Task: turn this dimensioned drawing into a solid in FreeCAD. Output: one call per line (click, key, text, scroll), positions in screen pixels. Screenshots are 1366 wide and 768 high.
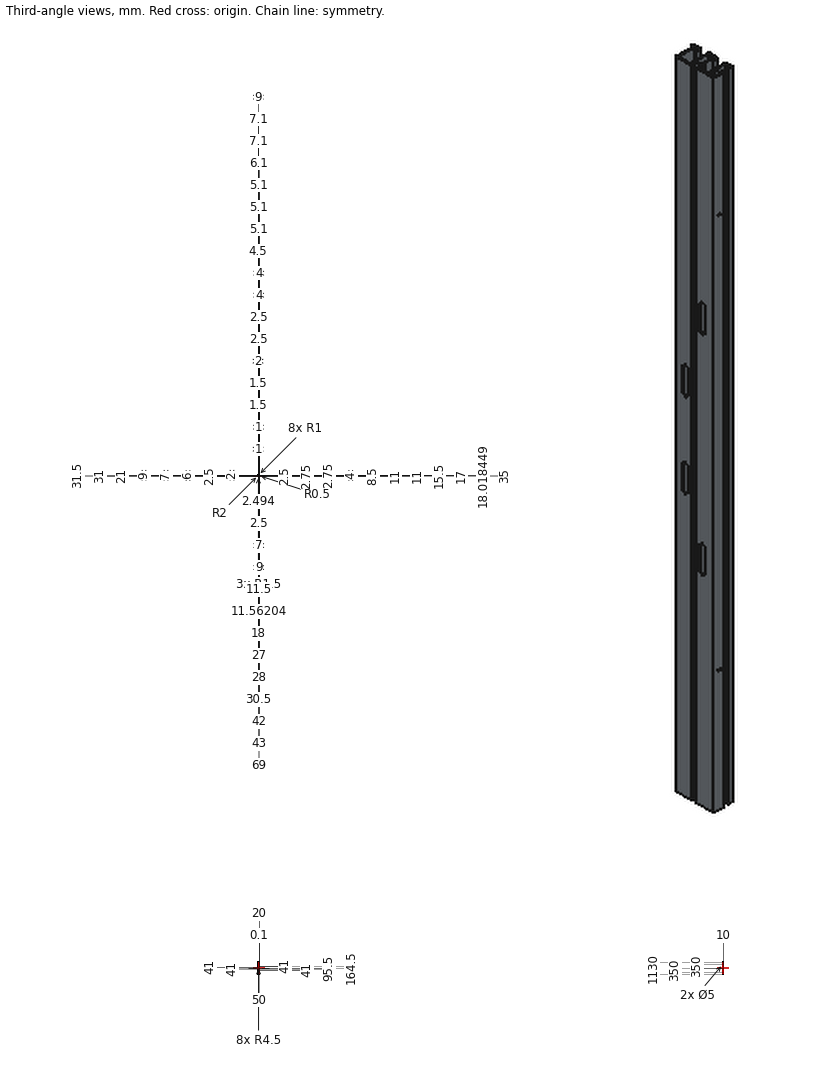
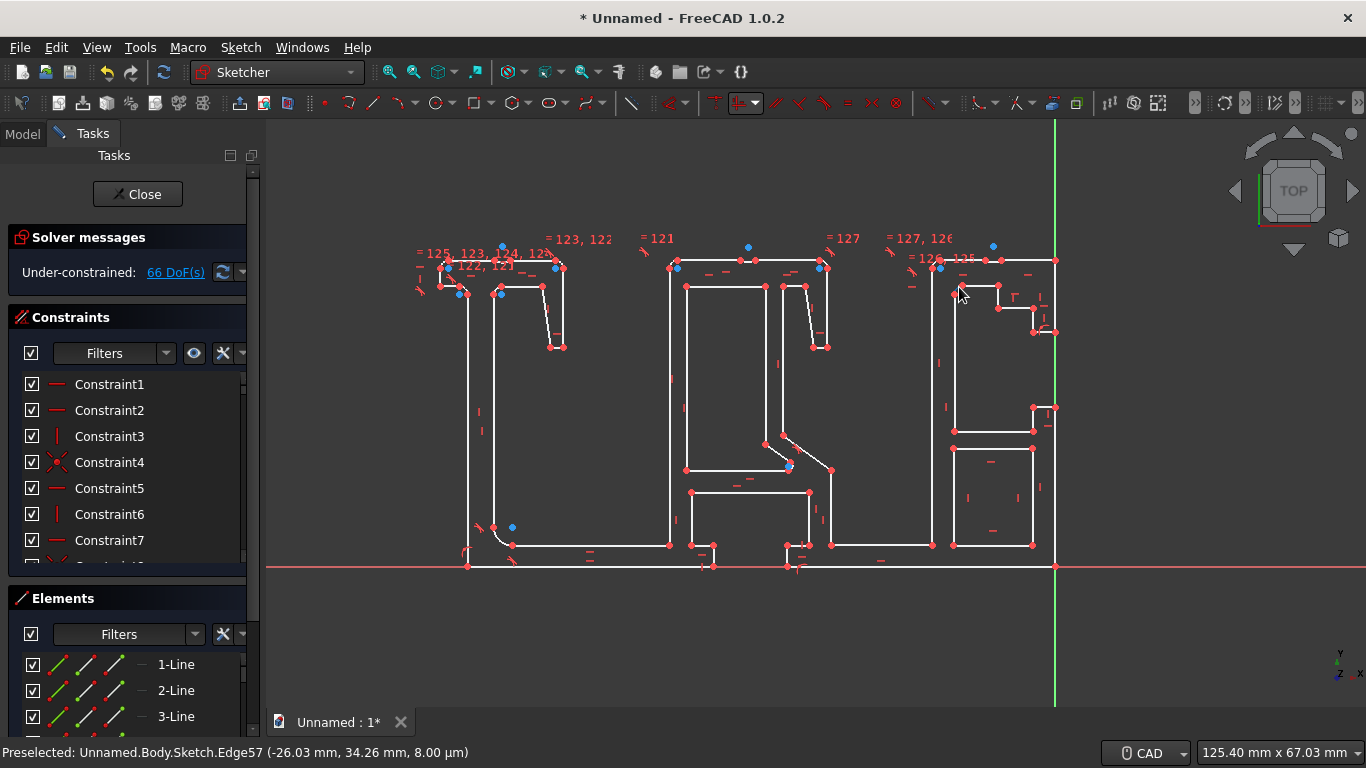
scroll(745, 262, up, 6)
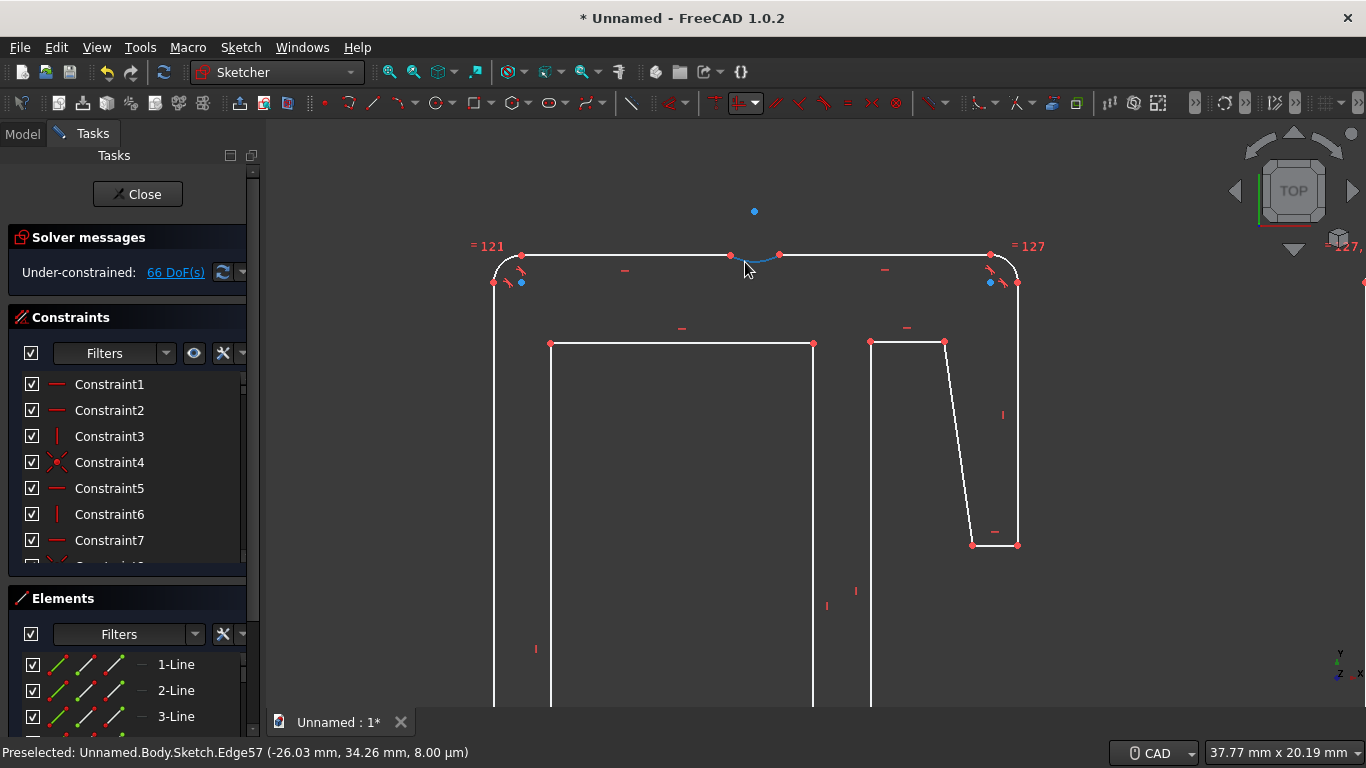
click(745, 261)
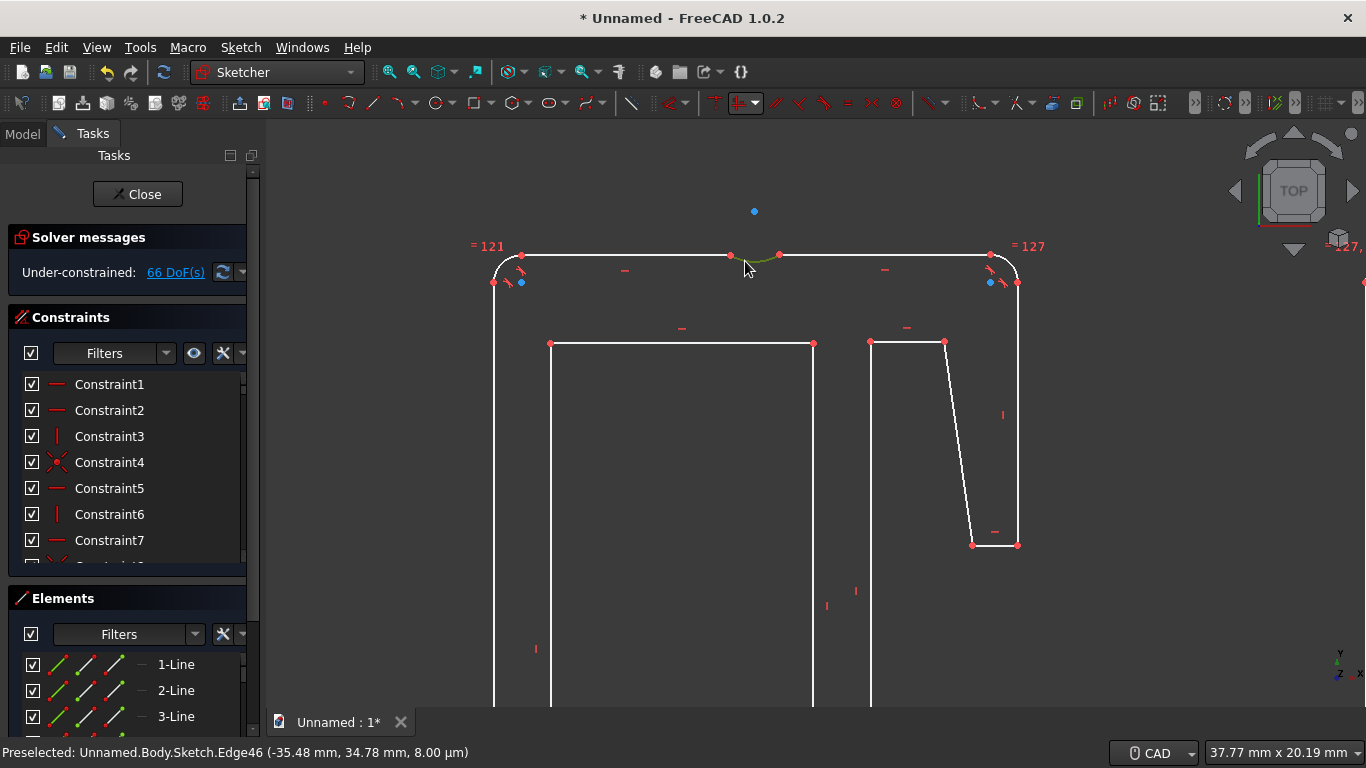
scroll(744, 262, down, 6)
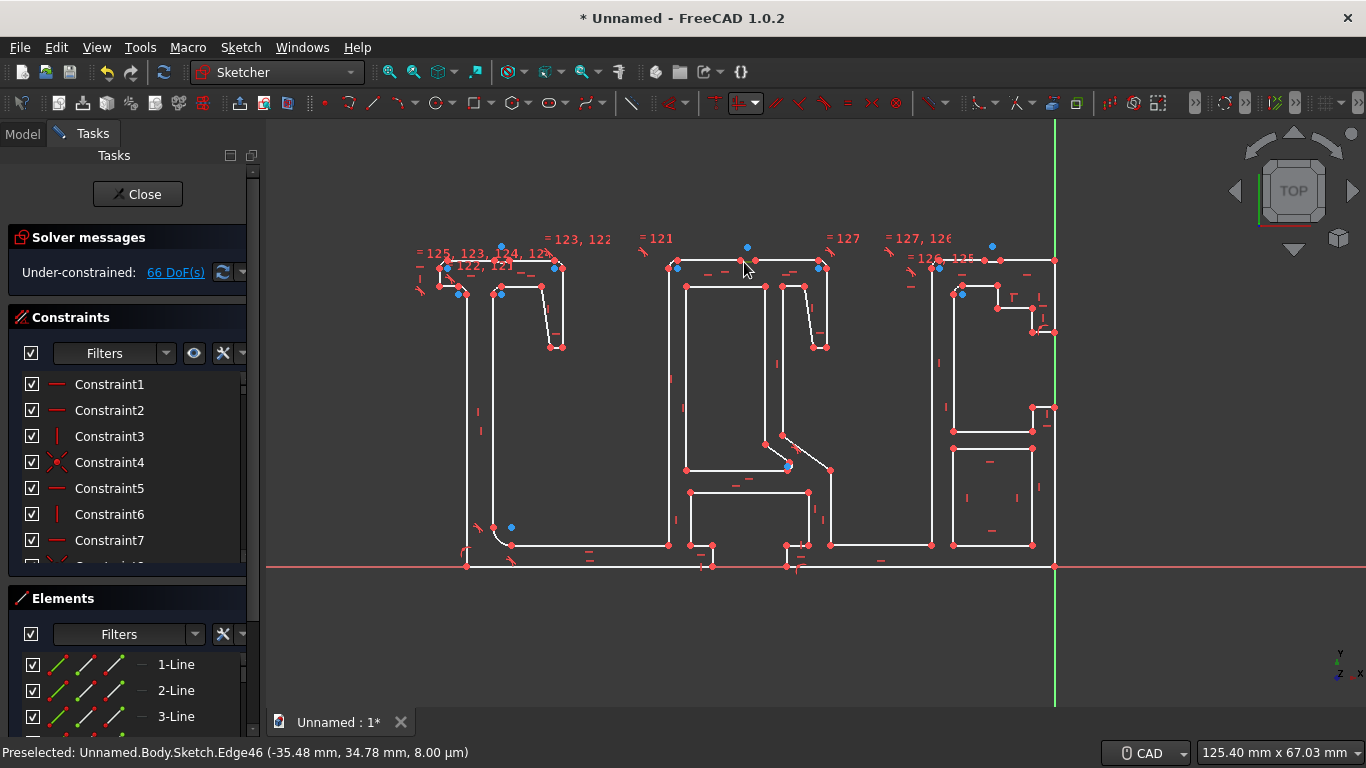
scroll(499, 262, up, 6)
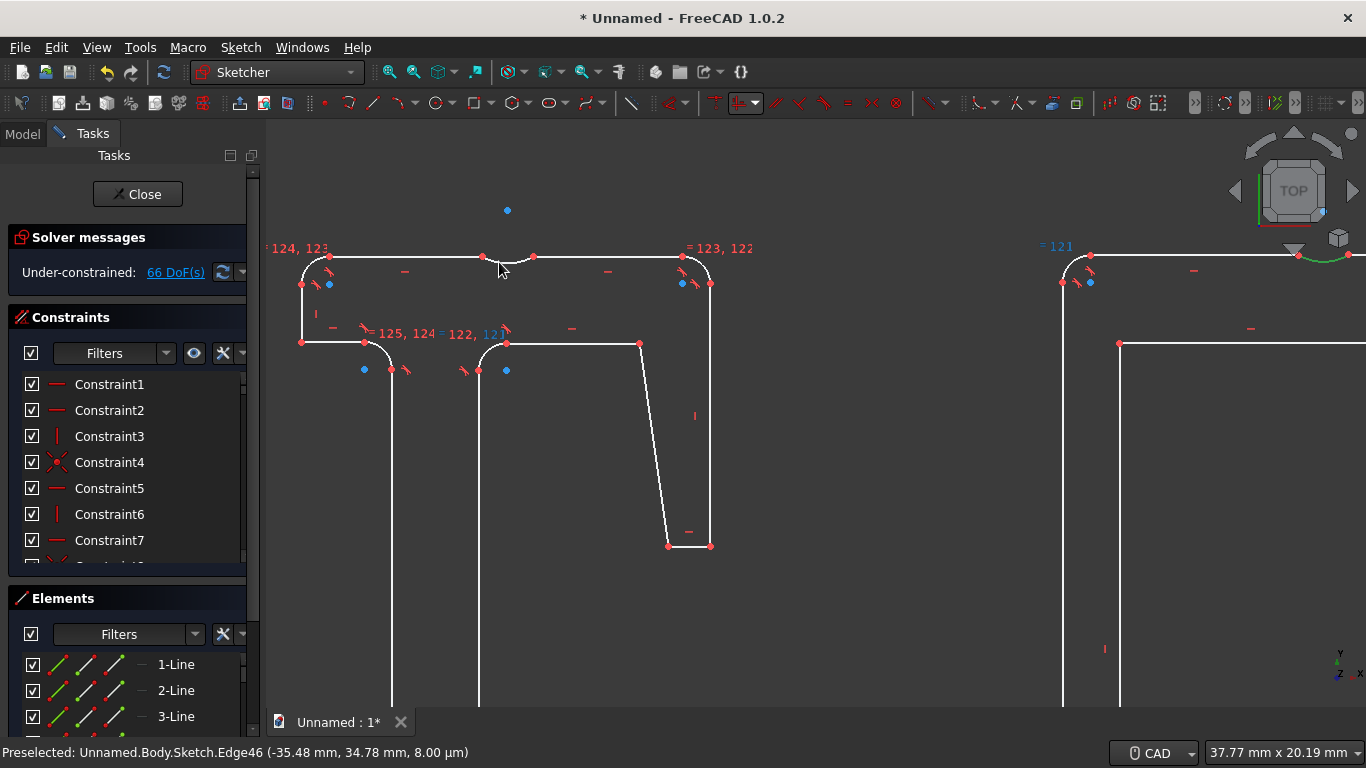
click(497, 262)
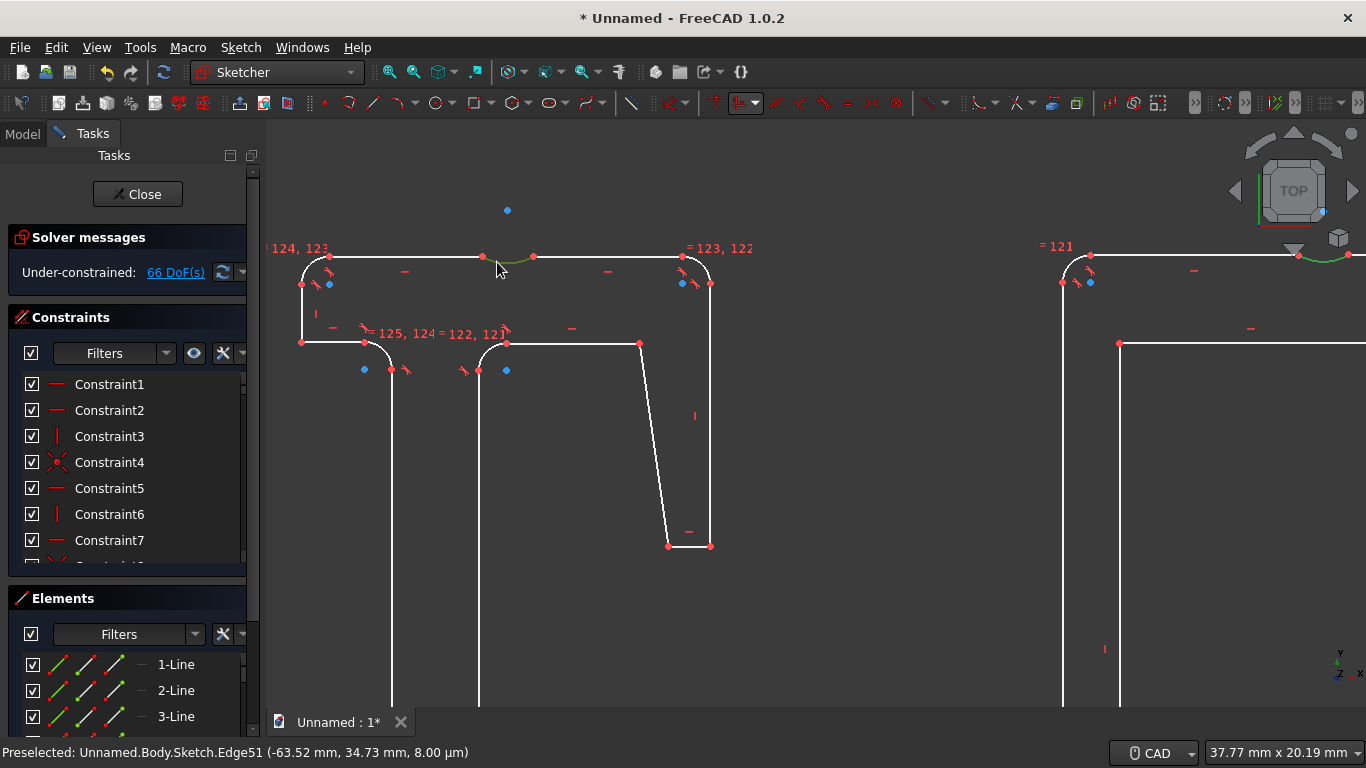
scroll(499, 262, down, 6)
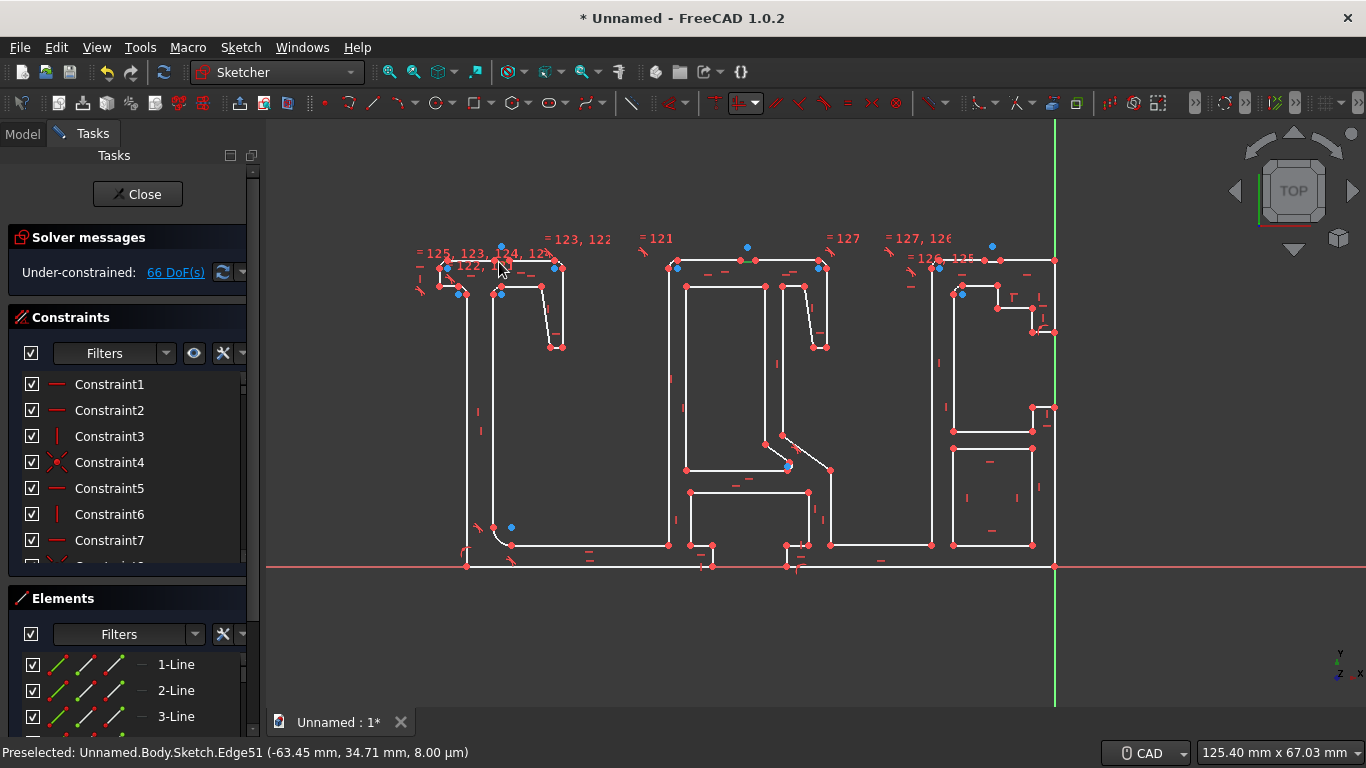
scroll(990, 262, up, 6)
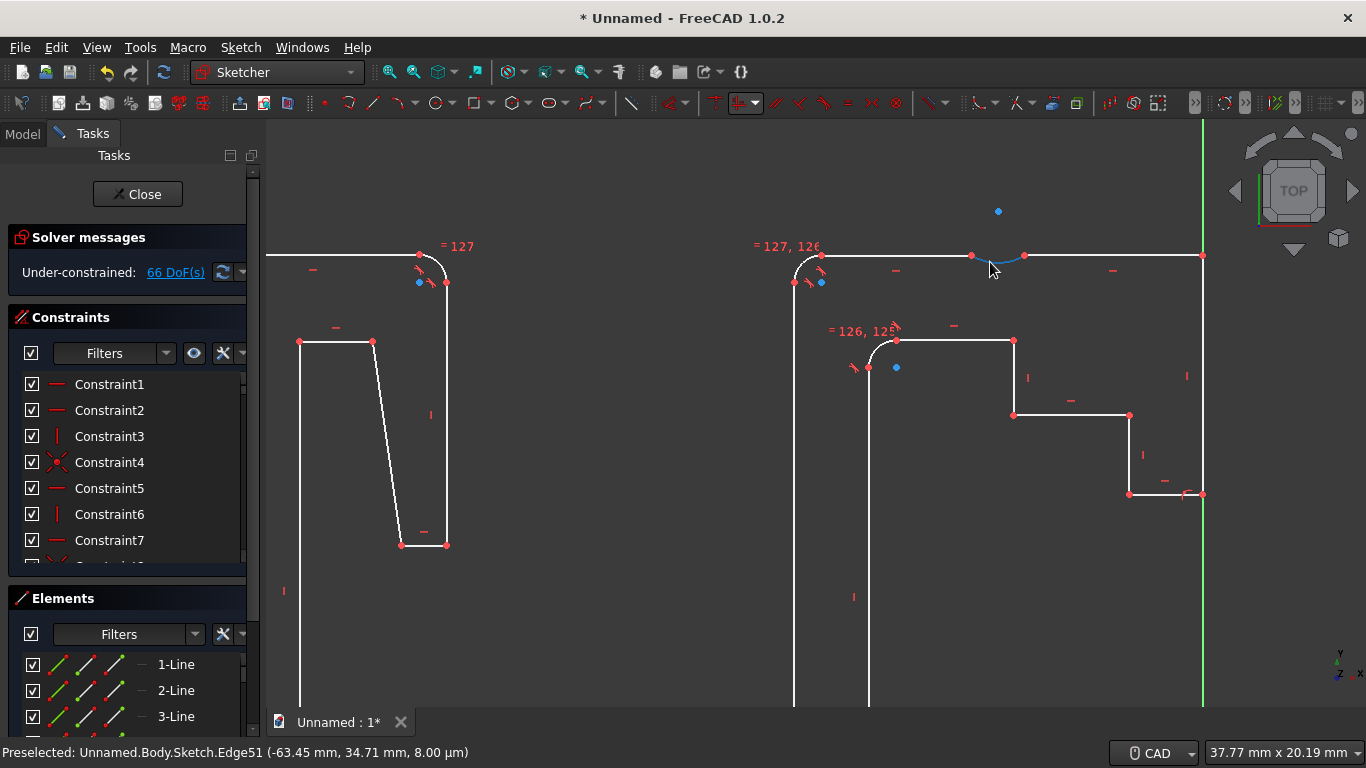
click(987, 262)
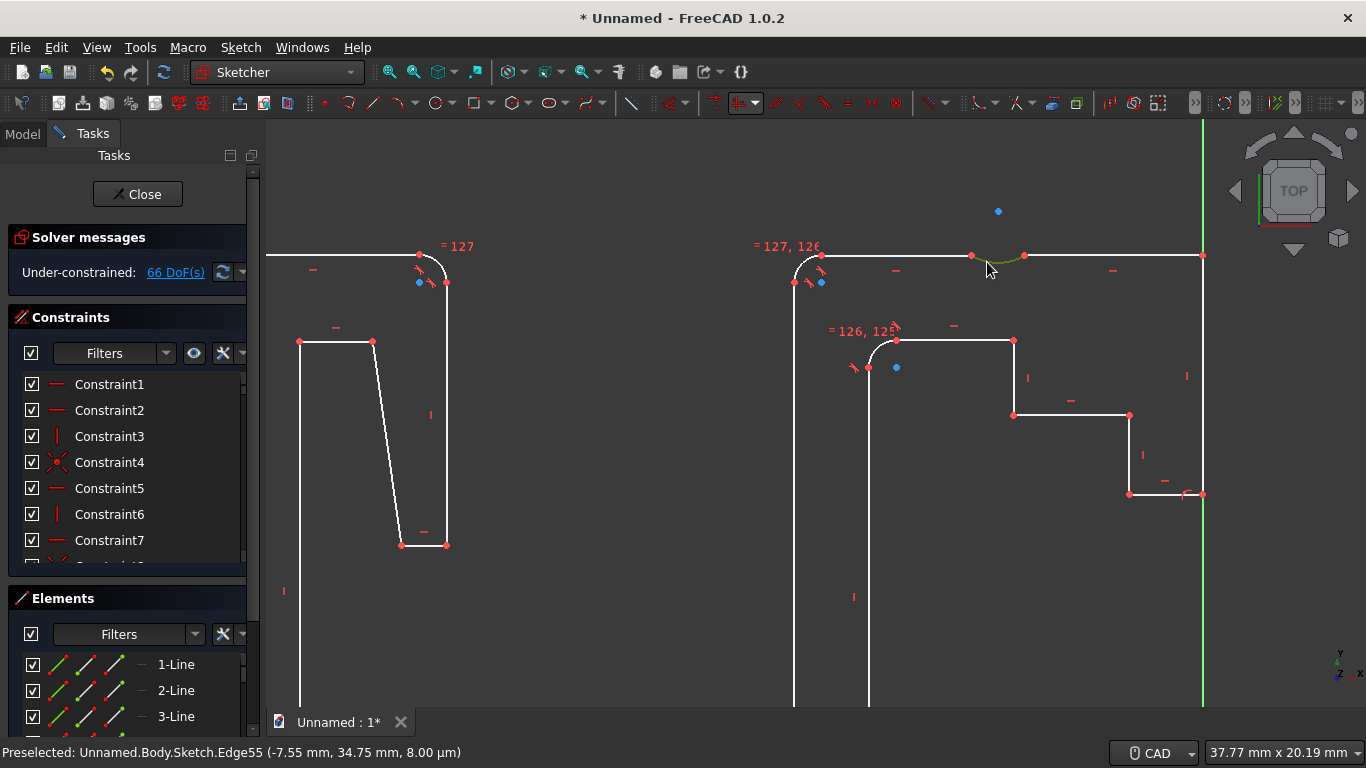
click(848, 104)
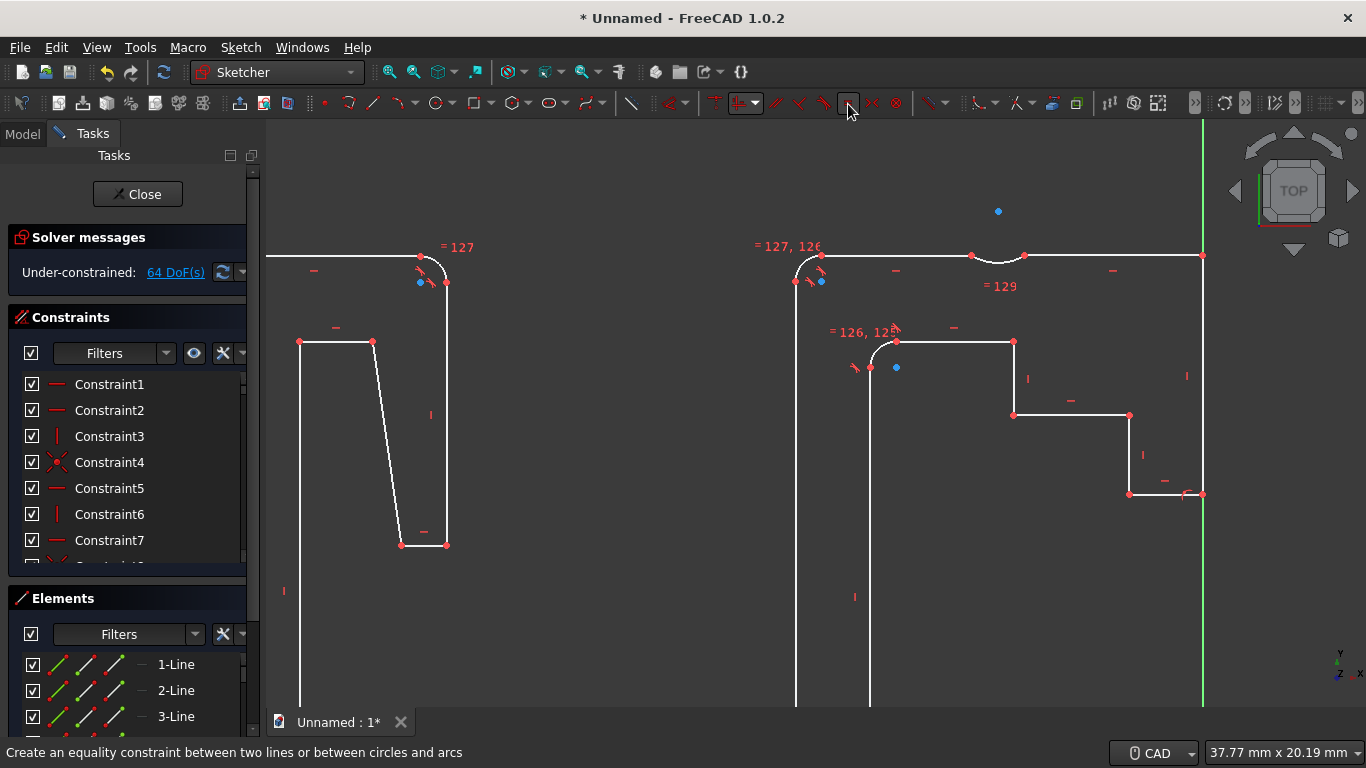
click(670, 104)